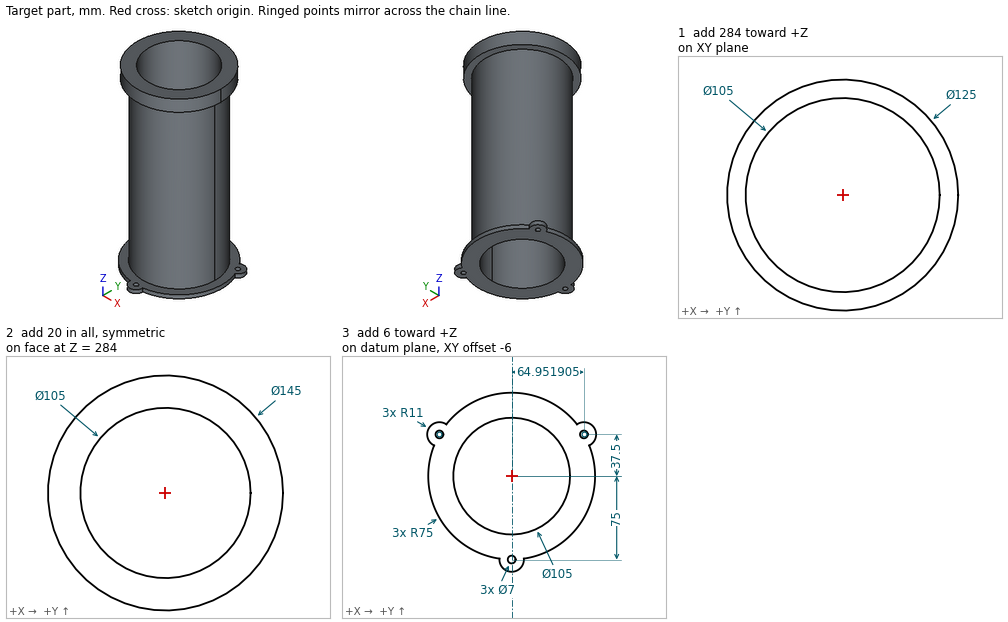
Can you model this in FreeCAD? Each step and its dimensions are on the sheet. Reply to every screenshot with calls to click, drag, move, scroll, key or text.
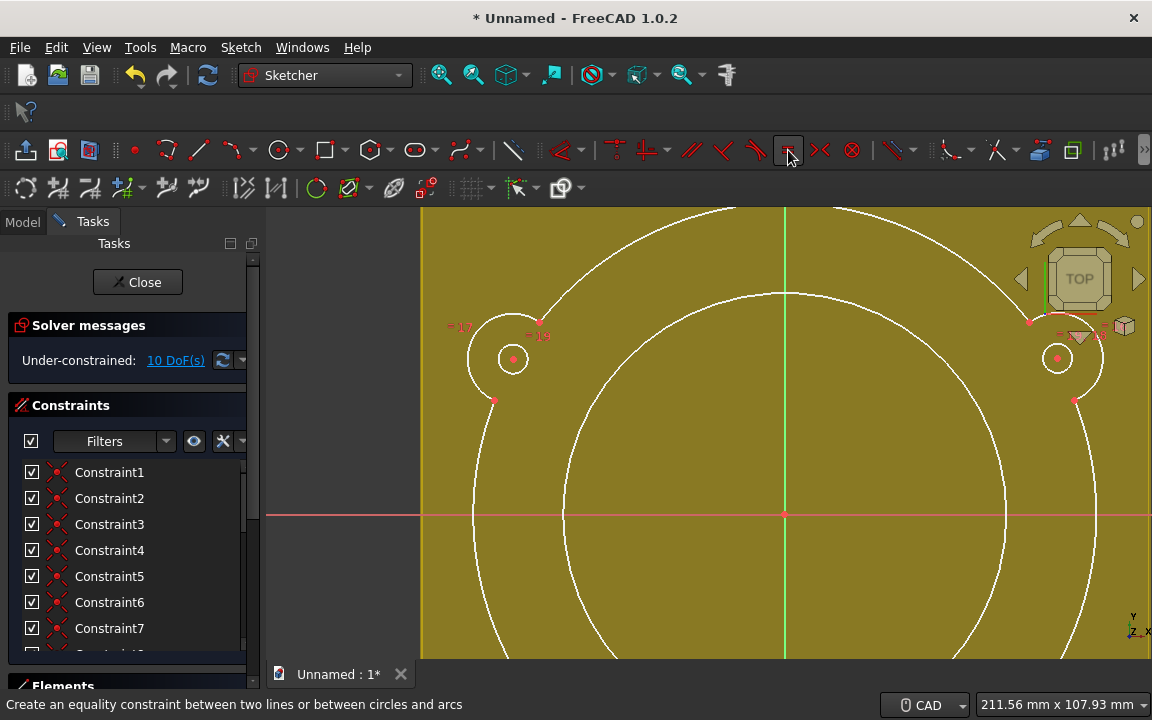
scroll(523, 348, down, 4)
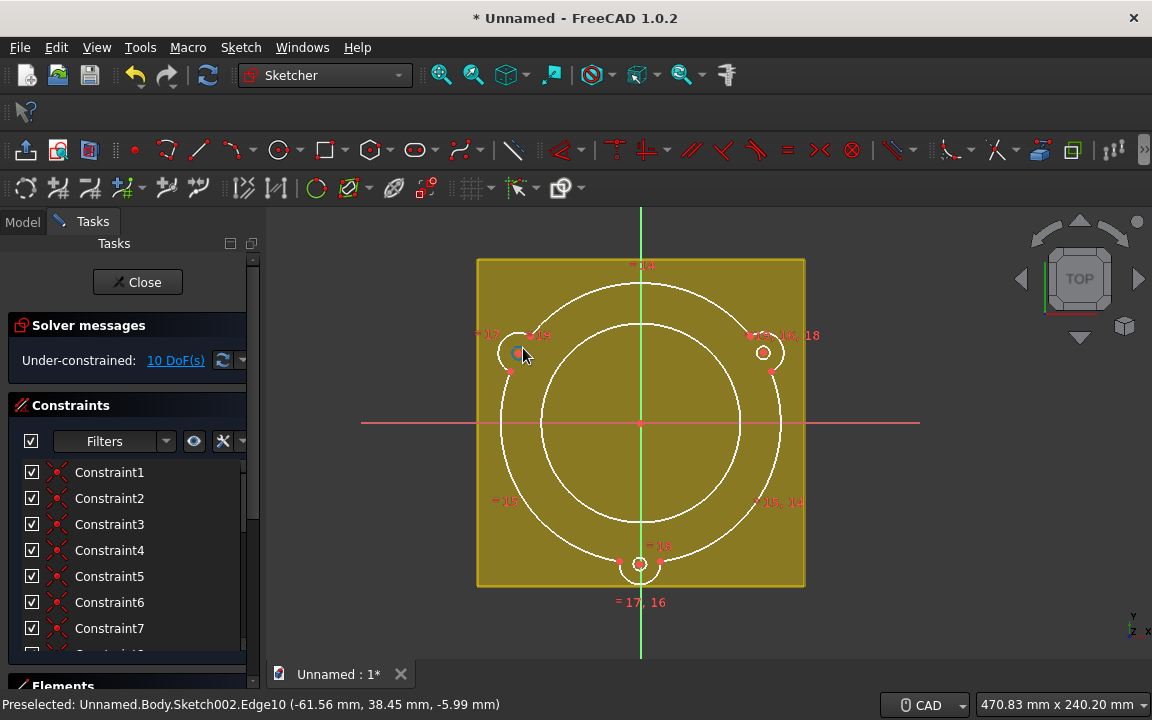
click(640, 564)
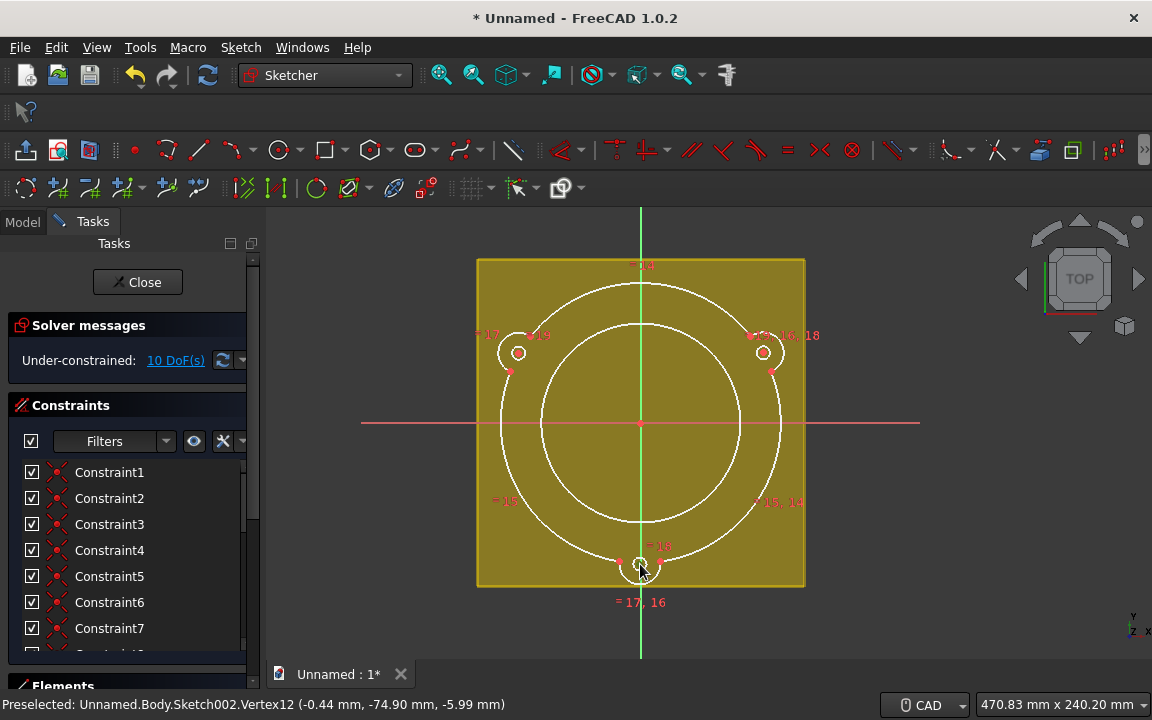
click(641, 490)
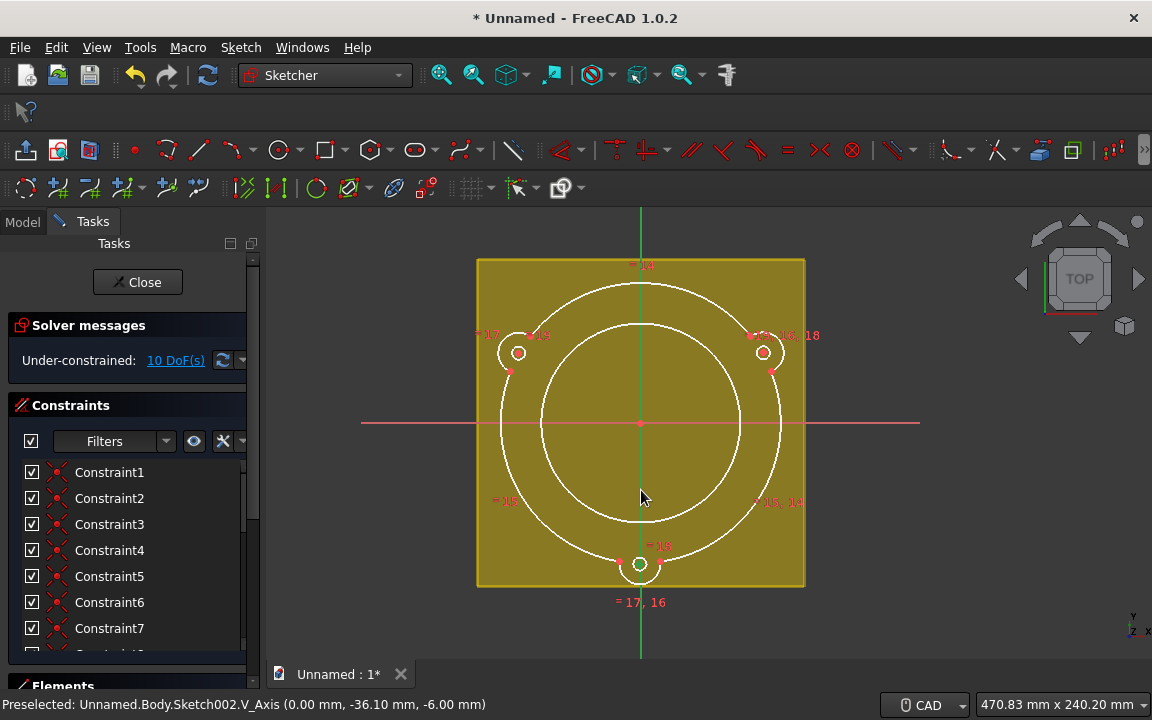
key(c)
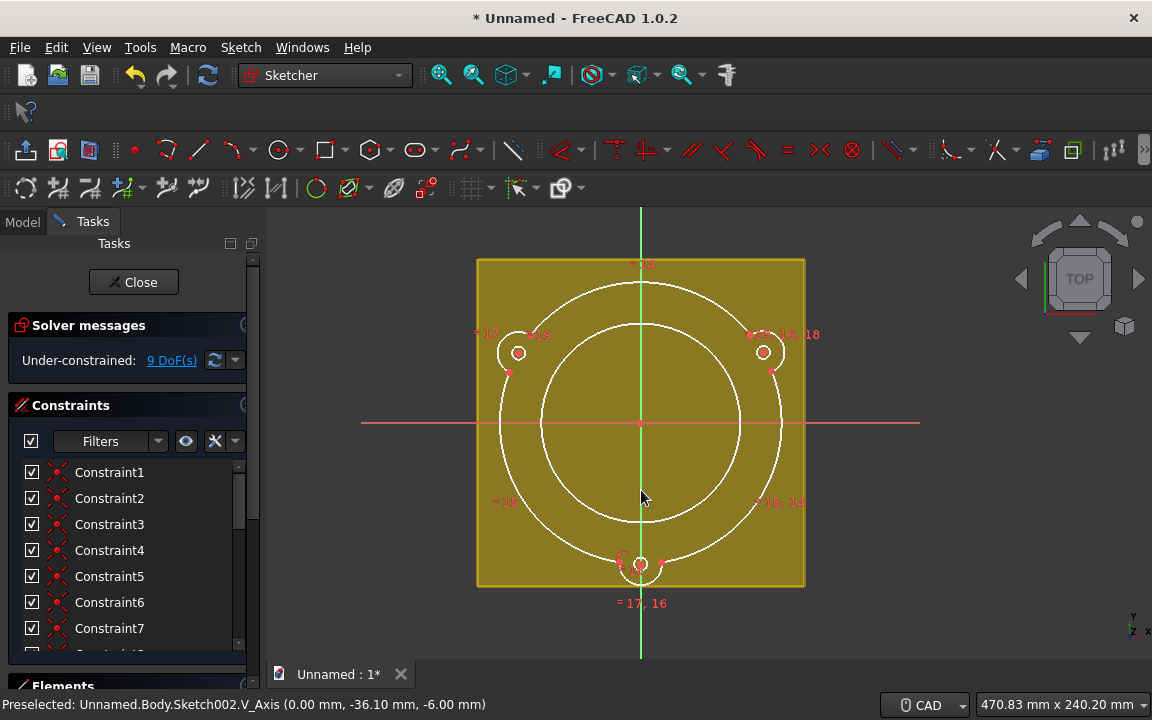
click(763, 352)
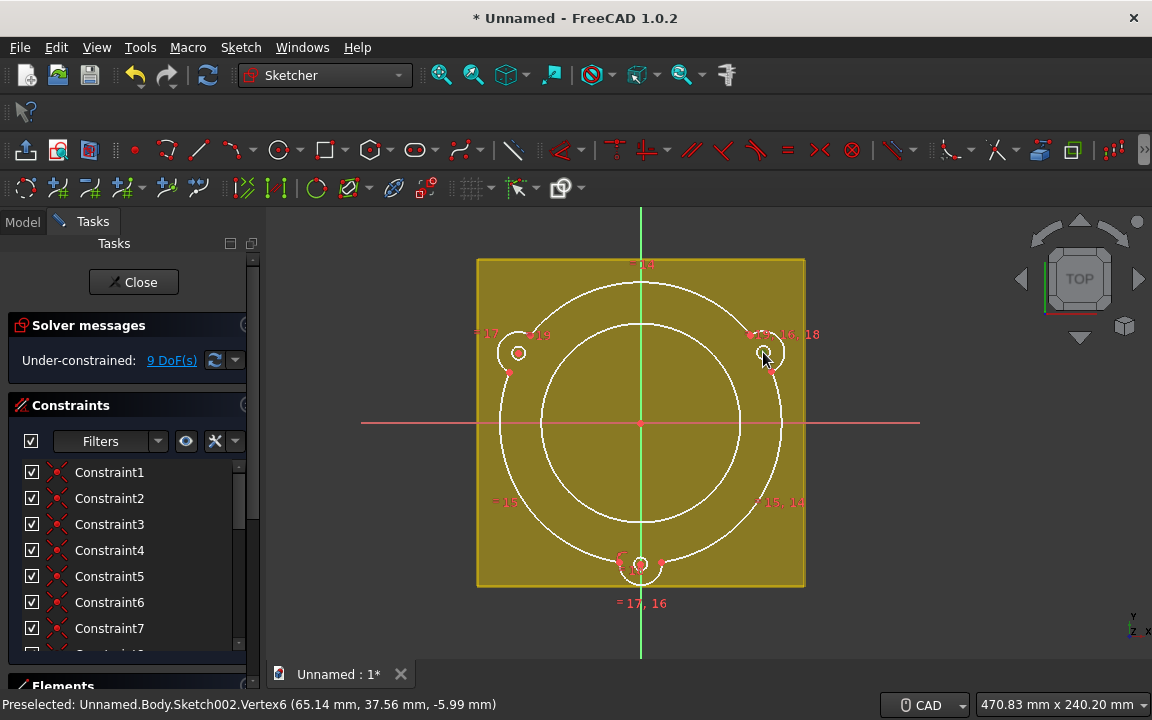
click(519, 353)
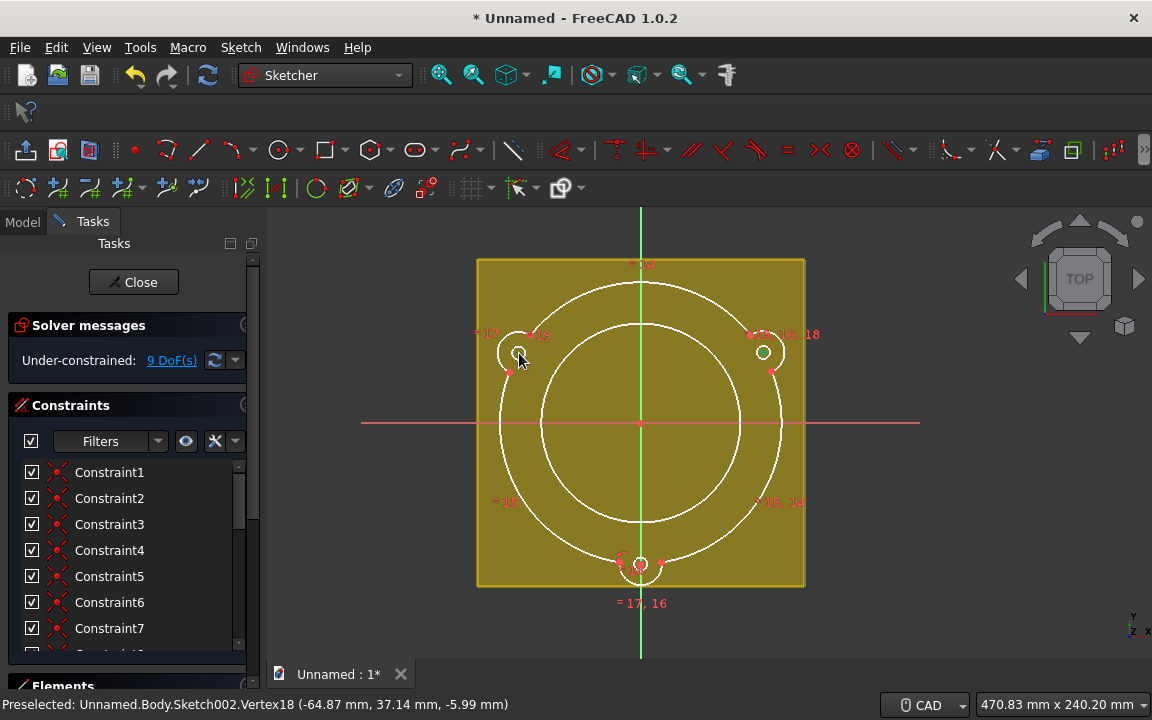
click(641, 490)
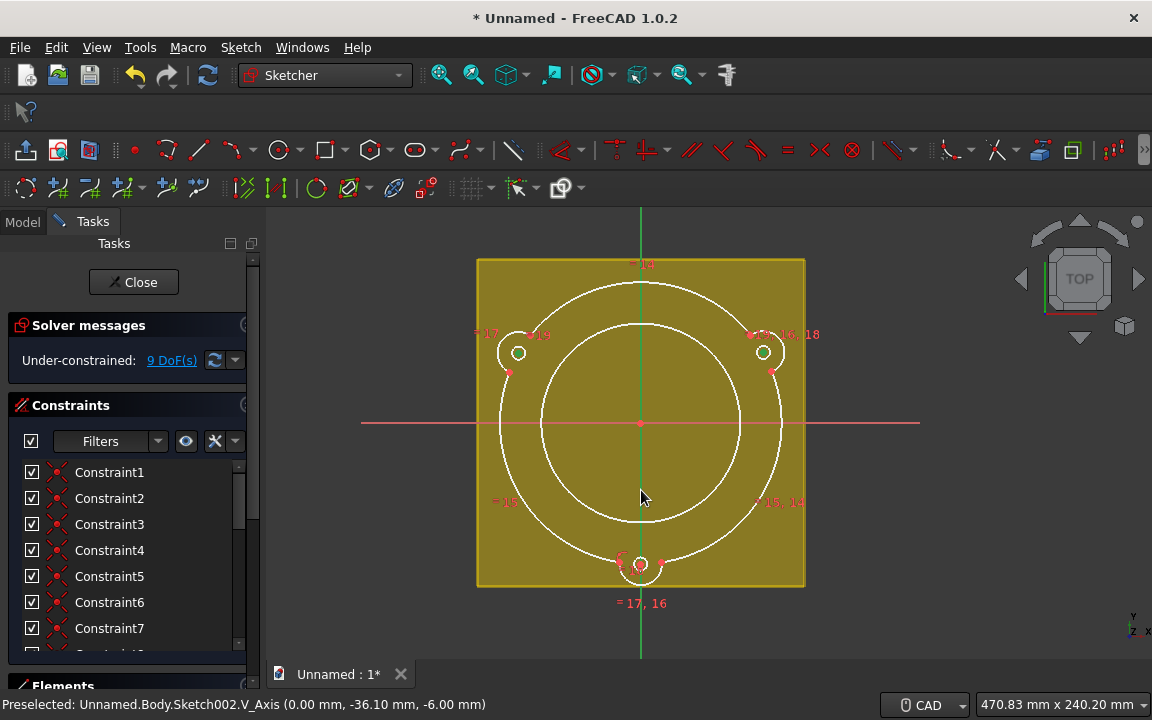
click(820, 150)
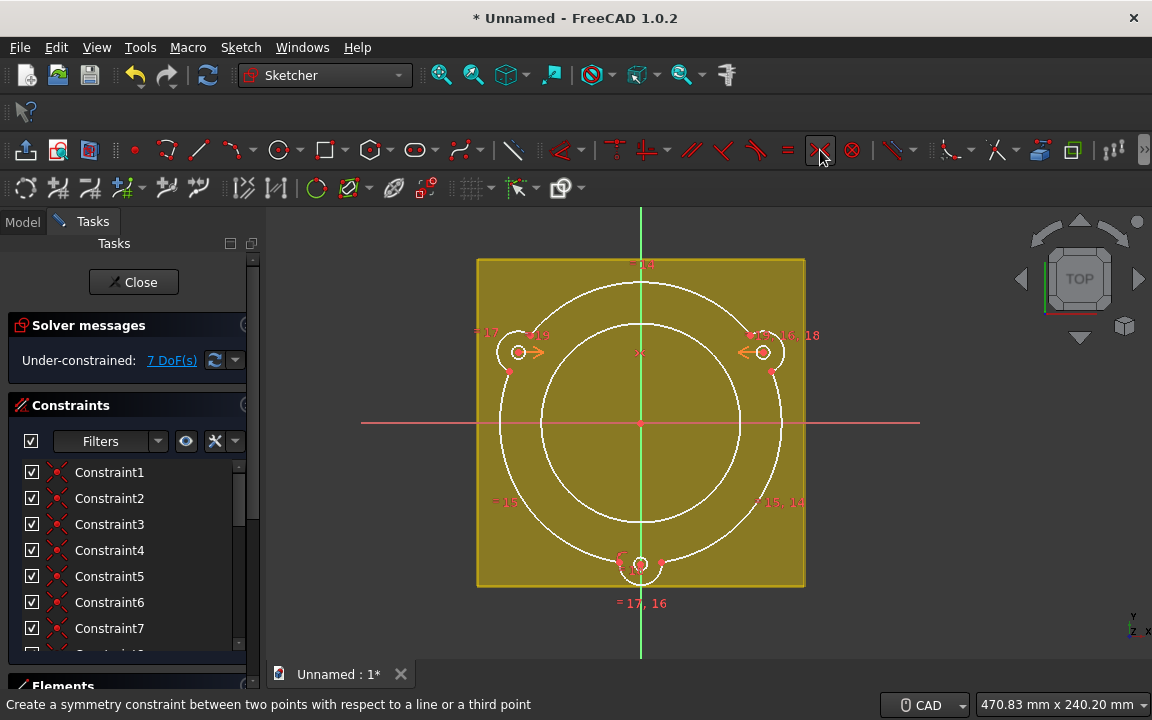
click(560, 150)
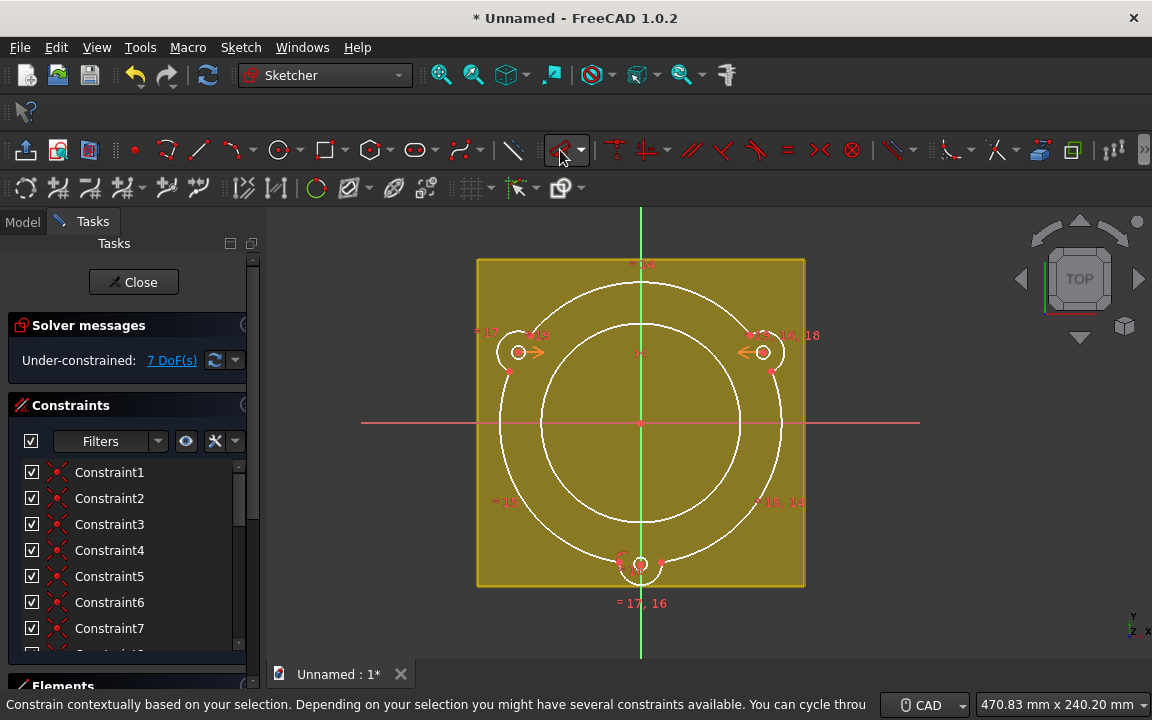
click(690, 291)
click(701, 261)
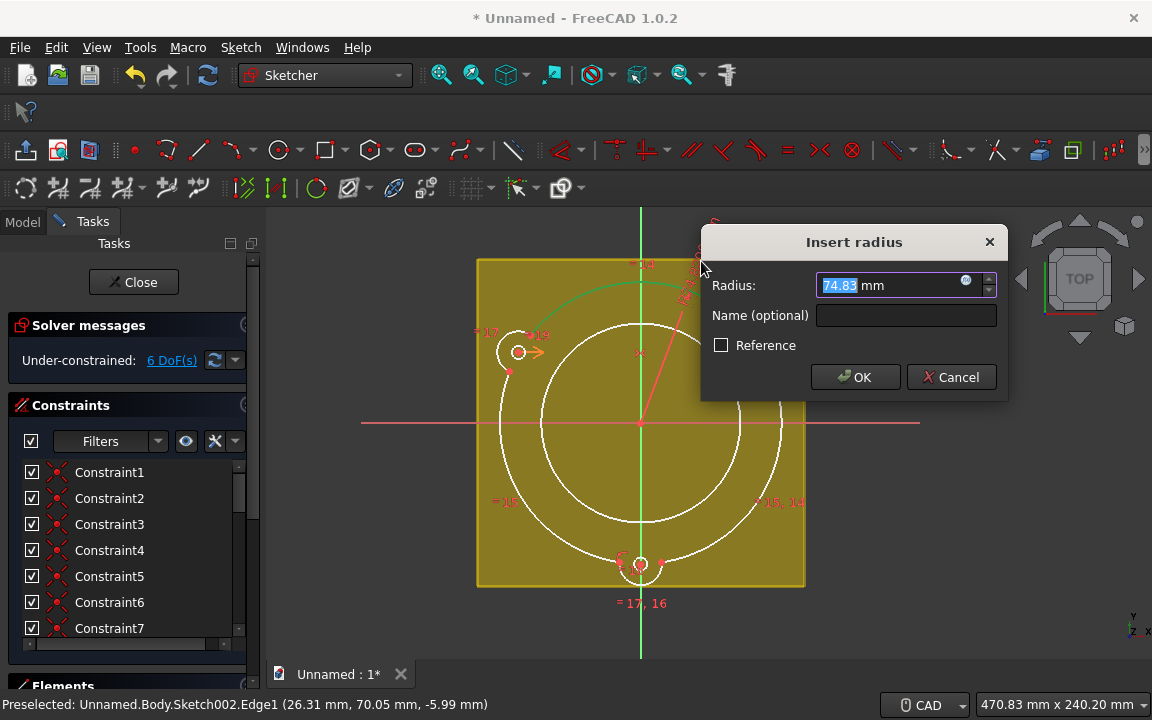
text(75)
key(Return)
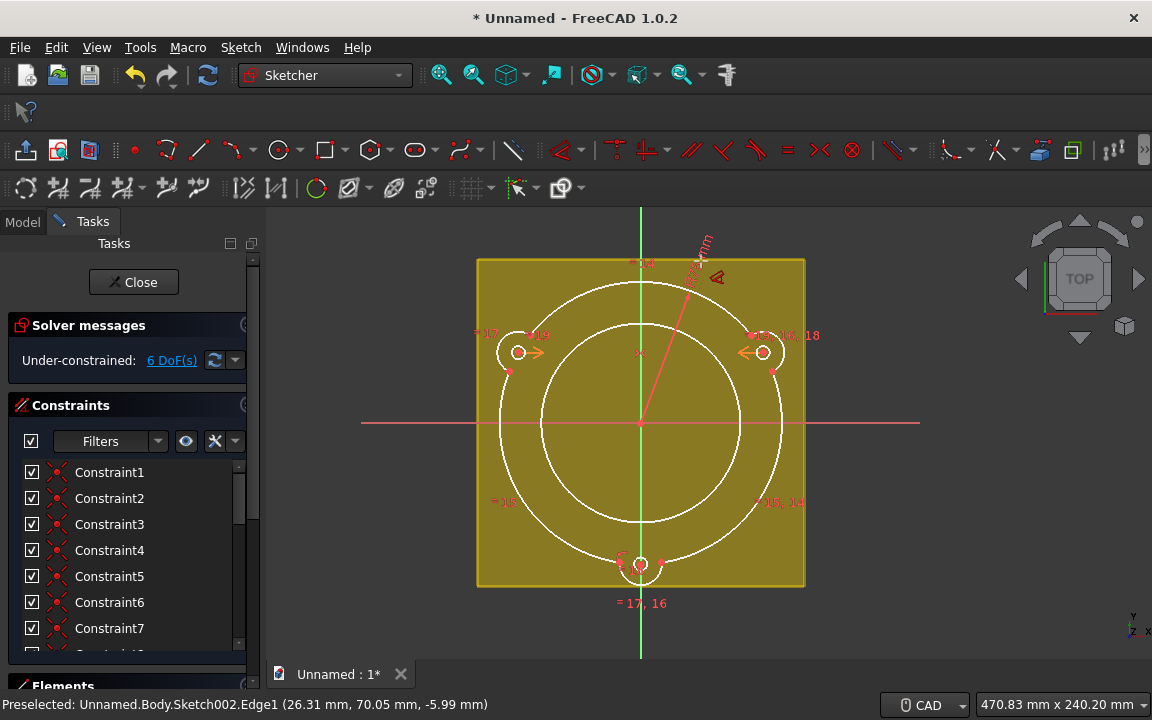
scroll(784, 356, up, 4)